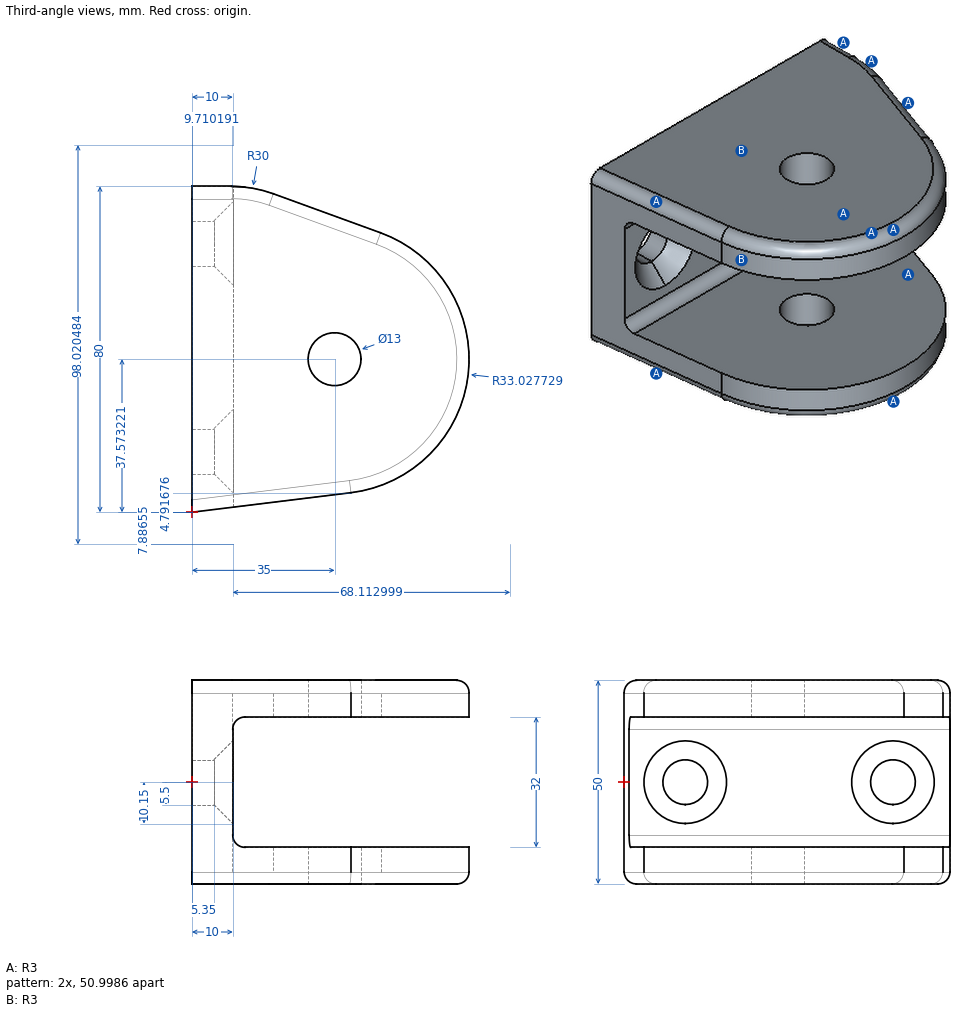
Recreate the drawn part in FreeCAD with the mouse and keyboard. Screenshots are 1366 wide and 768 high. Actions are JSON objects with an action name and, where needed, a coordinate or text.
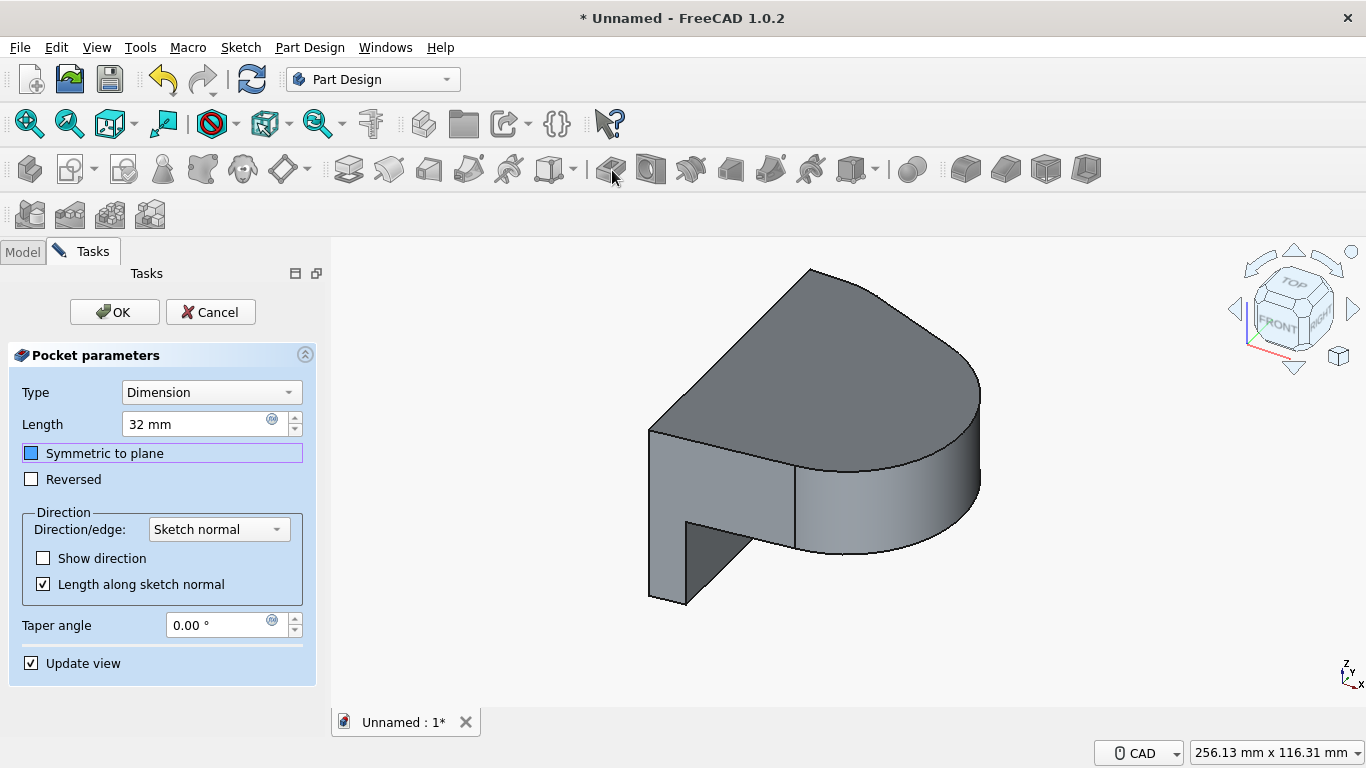
{"action": "left_click", "coordinate": [30, 453]}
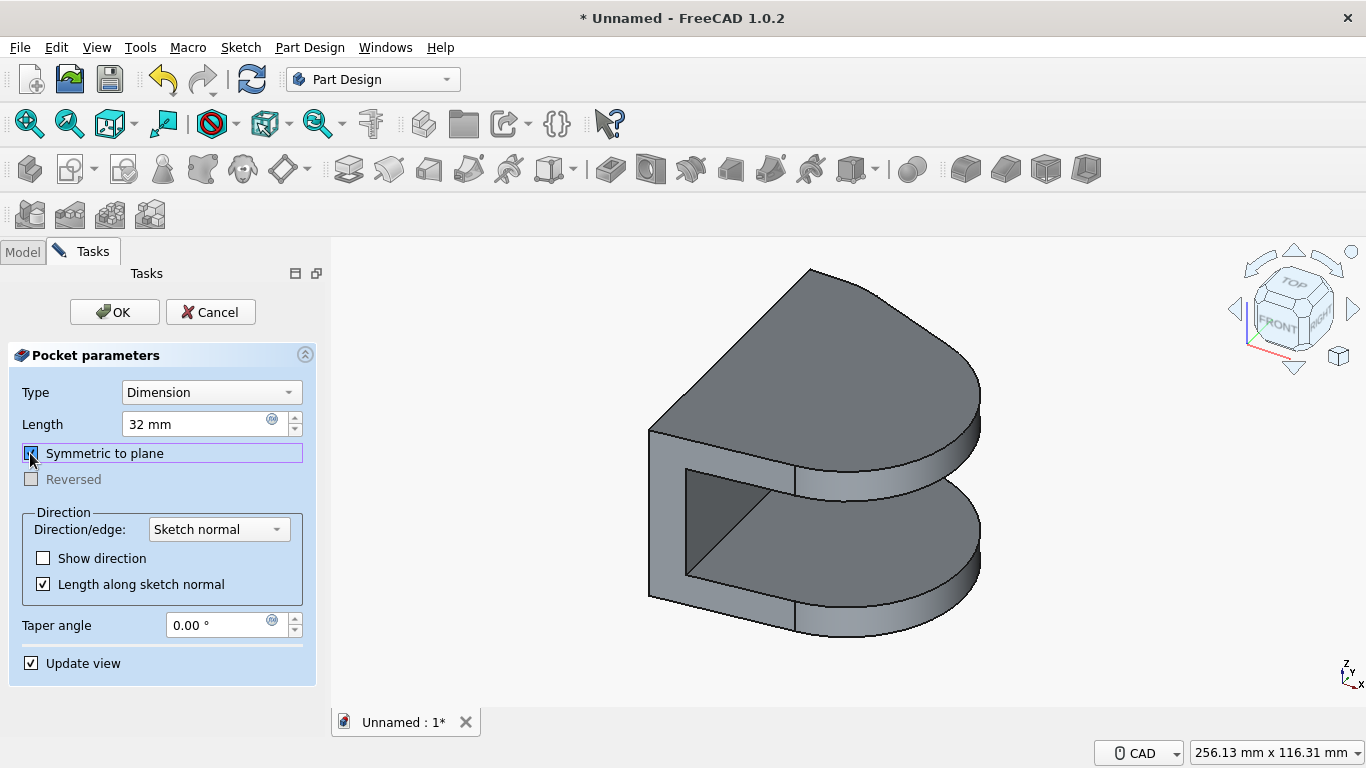
{"action": "left_click", "coordinate": [115, 312]}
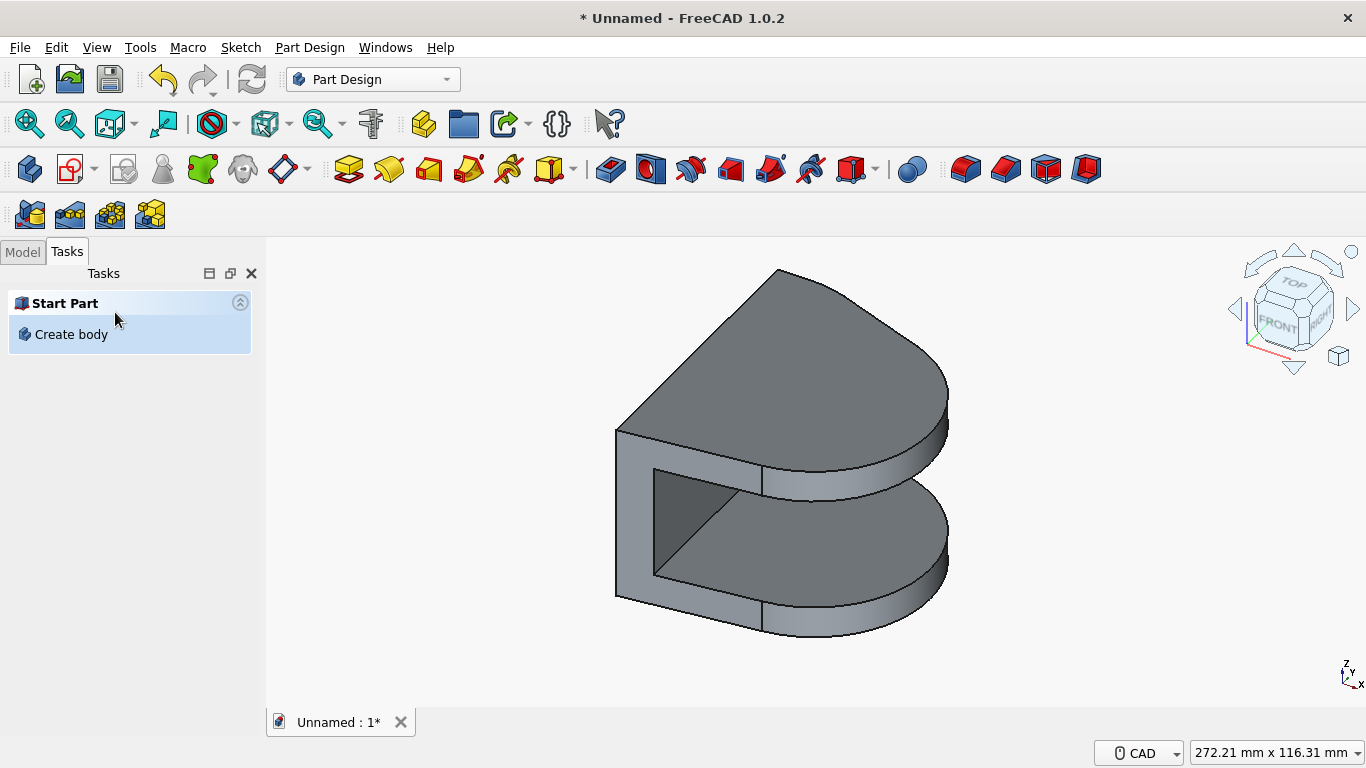
{"action": "left_click", "coordinate": [816, 388]}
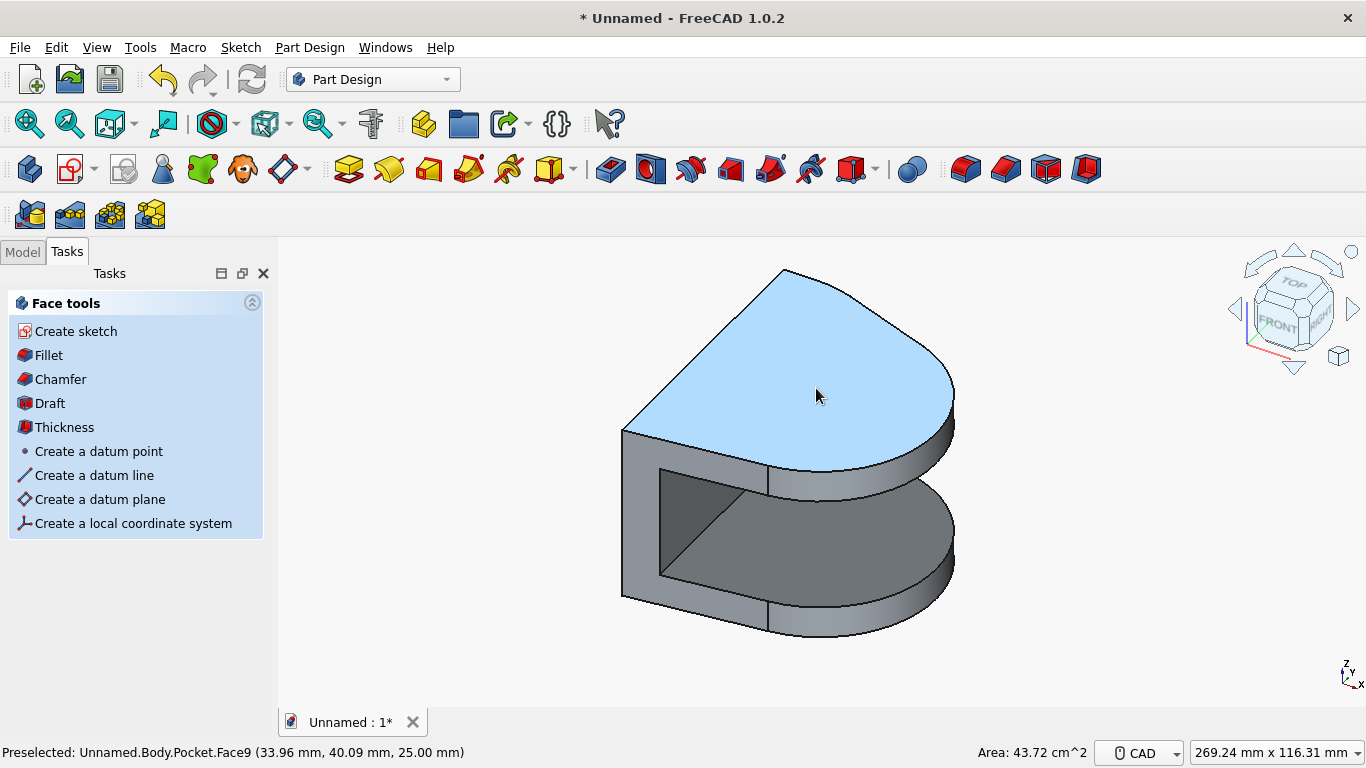
{"action": "left_click", "coordinate": [70, 170]}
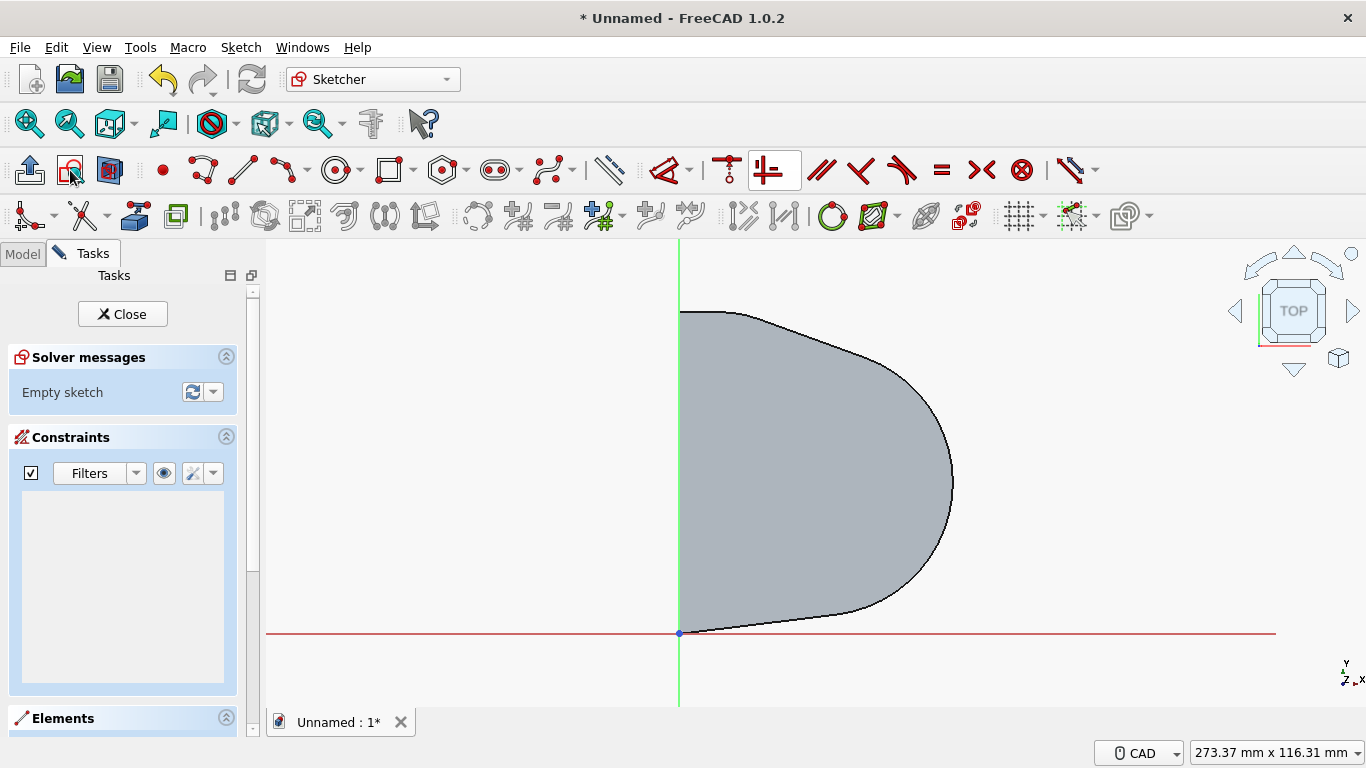
{"action": "scroll", "coordinate": [834, 485], "scroll_direction": "up", "scroll_amount": 9}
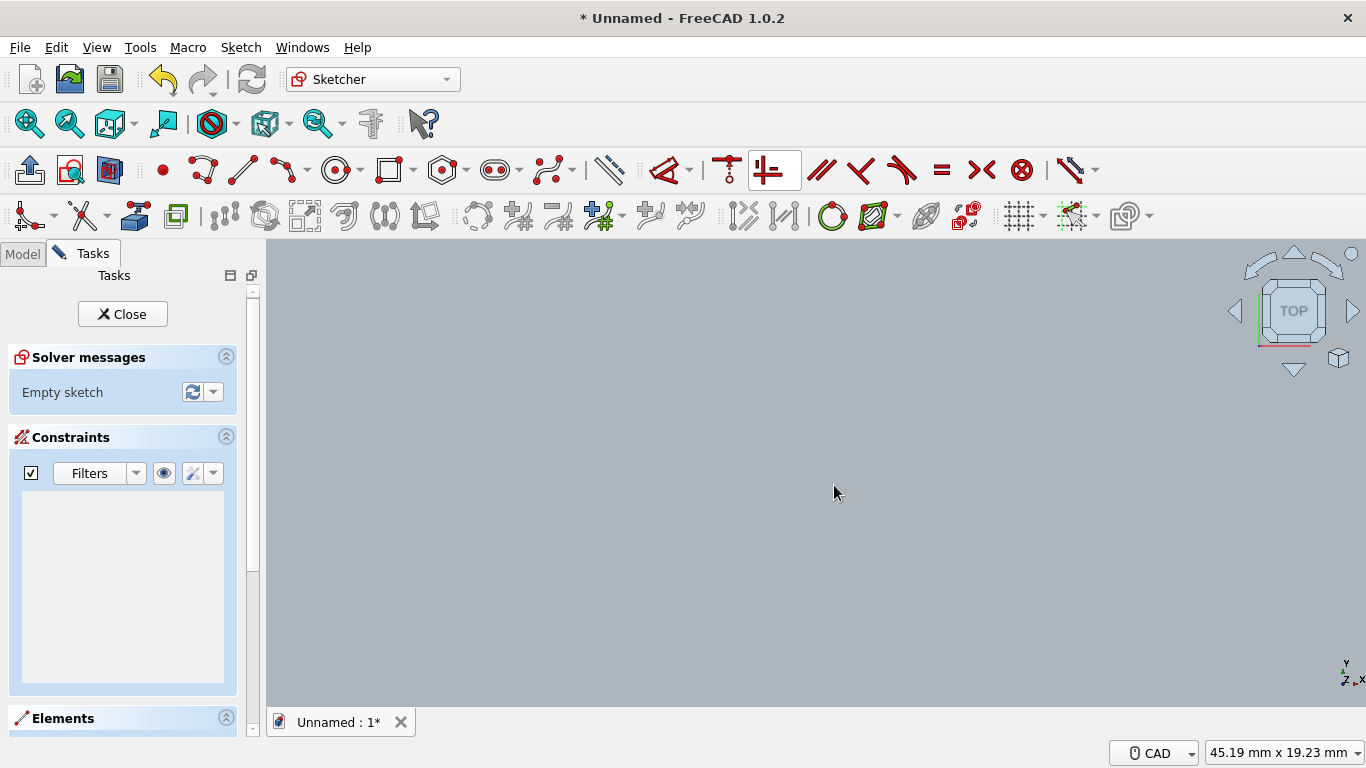
{"action": "left_click", "coordinate": [336, 170]}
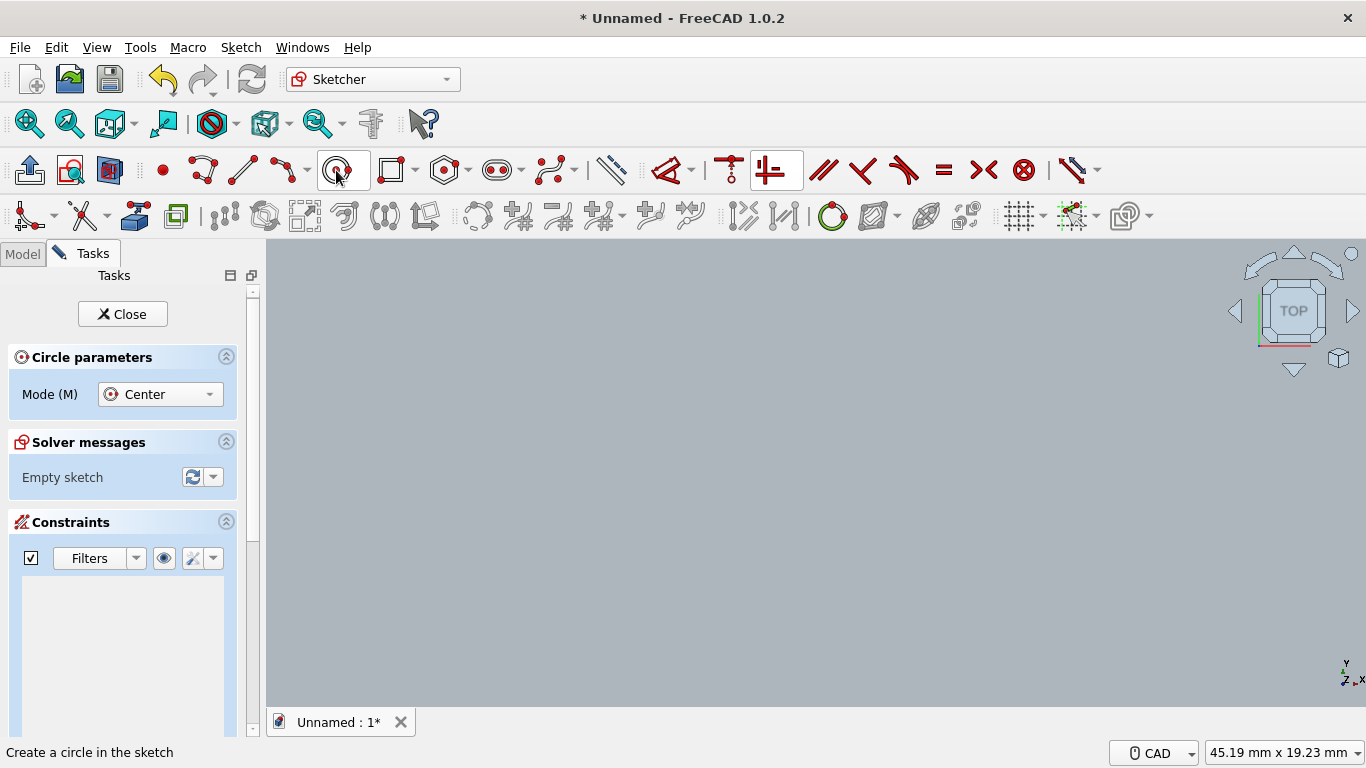
{"action": "left_click", "coordinate": [747, 469]}
{"action": "left_click", "coordinate": [858, 357]}
{"action": "key", "text": "Escape"}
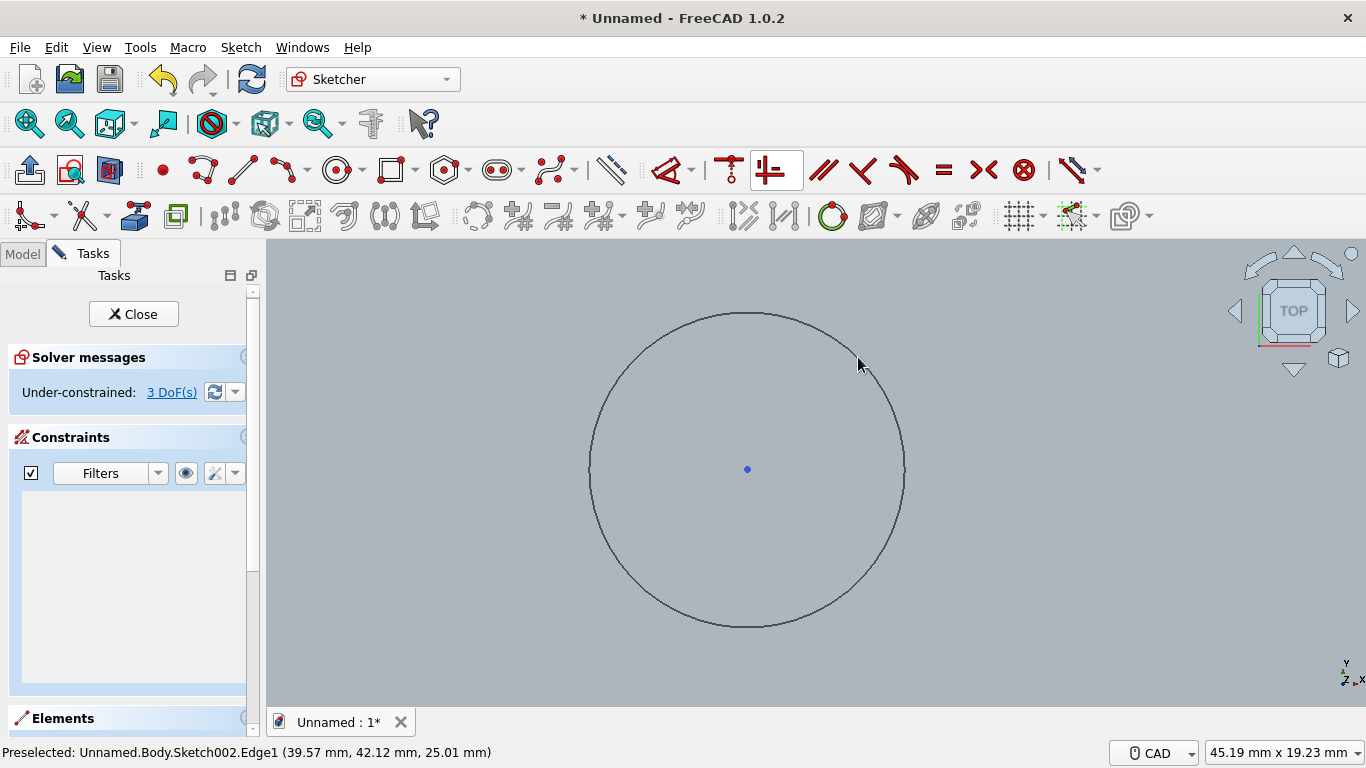
{"action": "left_click", "coordinate": [666, 170]}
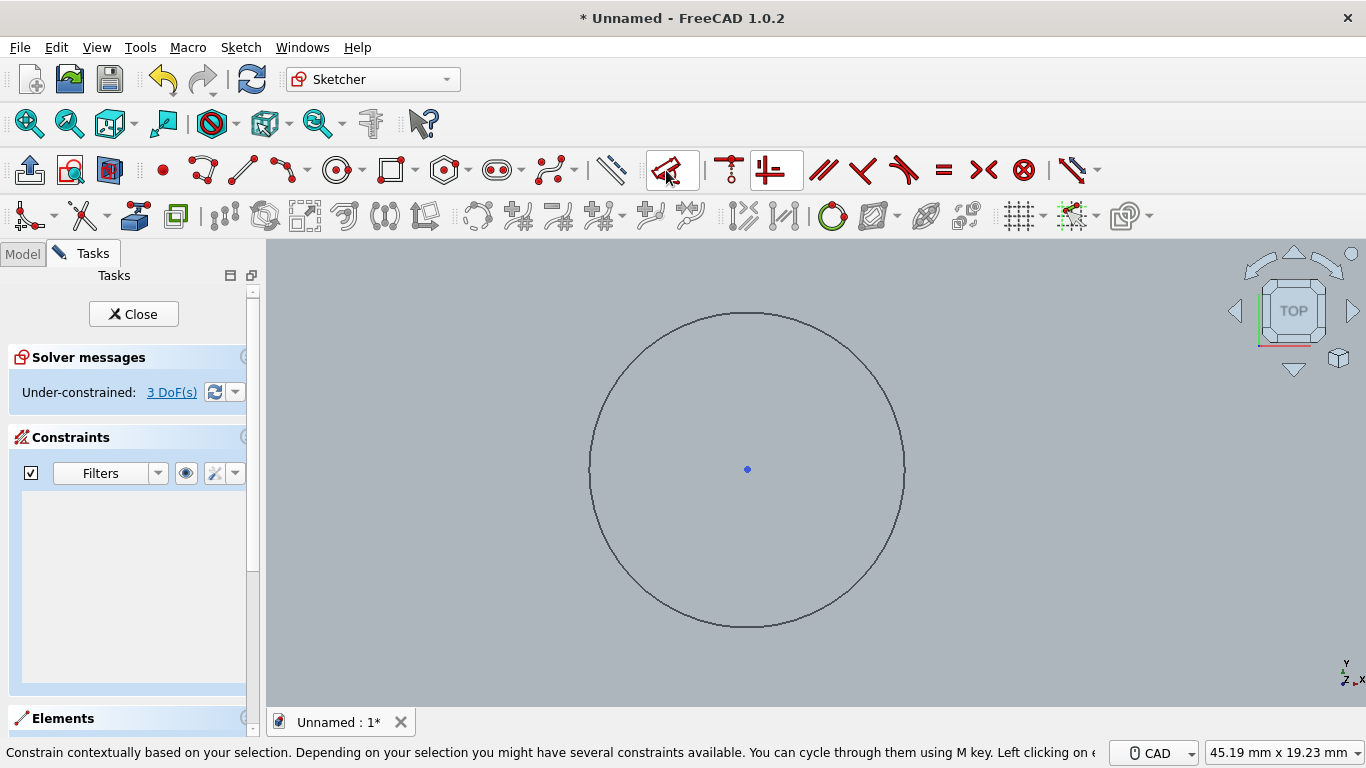
{"action": "left_click", "coordinate": [858, 358]}
{"action": "left_click", "coordinate": [881, 335]}